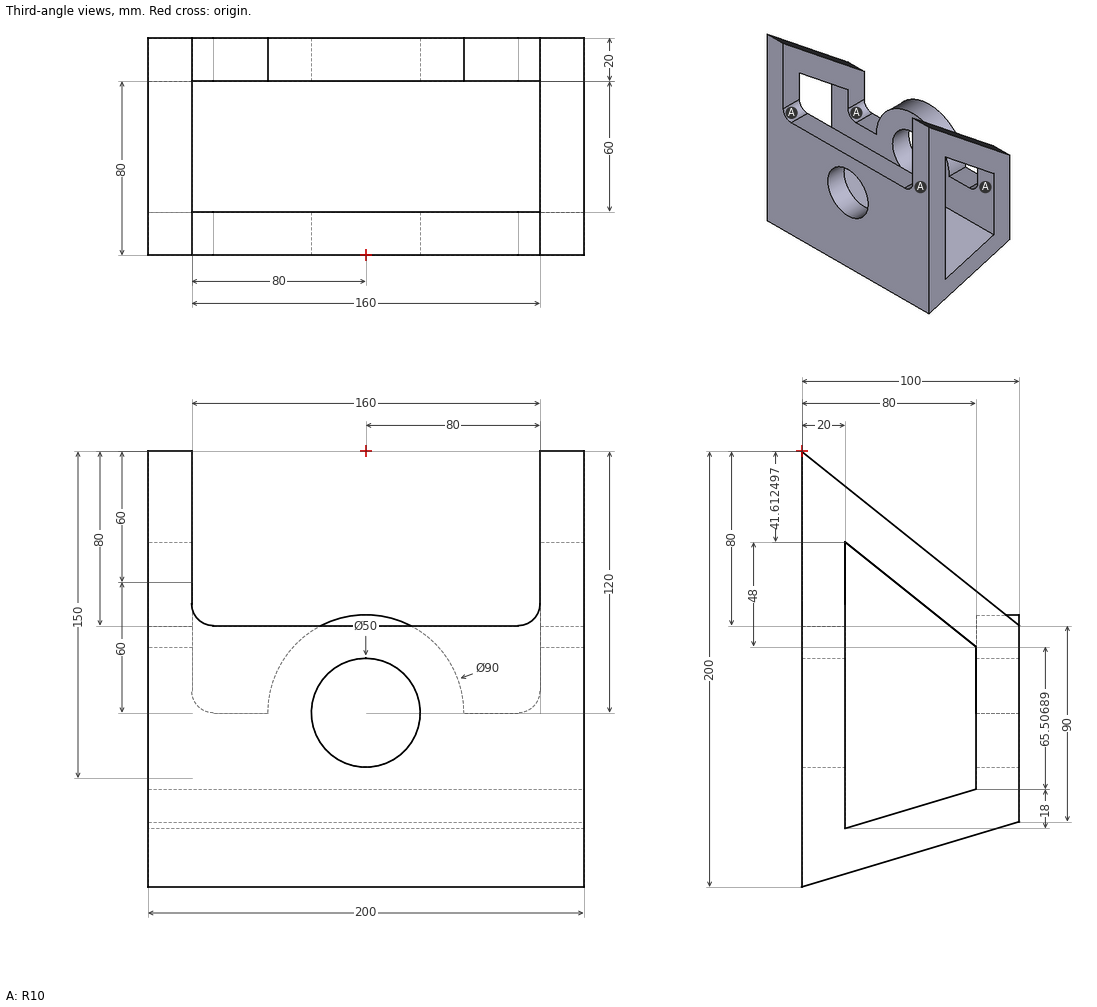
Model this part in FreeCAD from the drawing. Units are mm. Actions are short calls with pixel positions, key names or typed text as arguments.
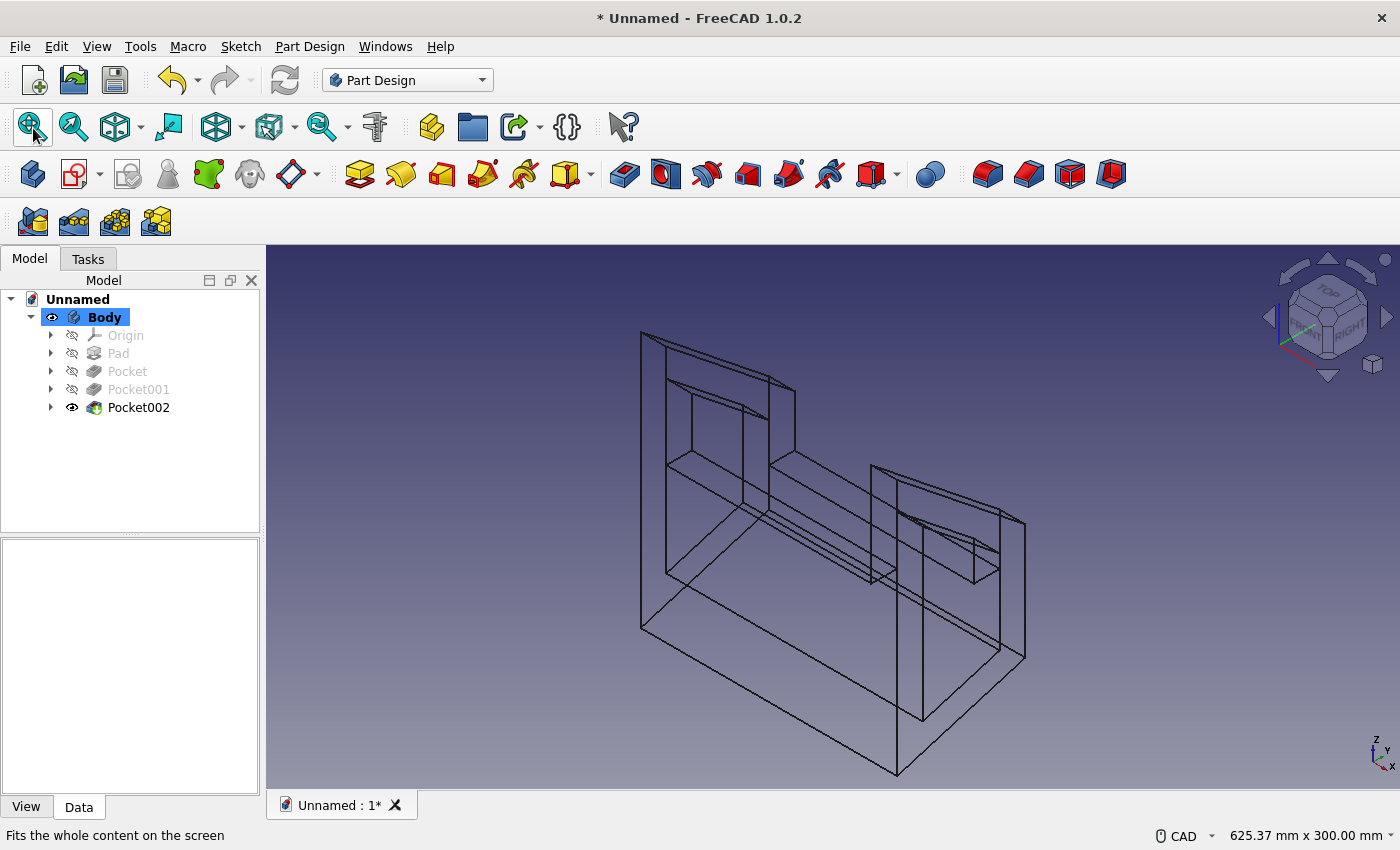
click(987, 575)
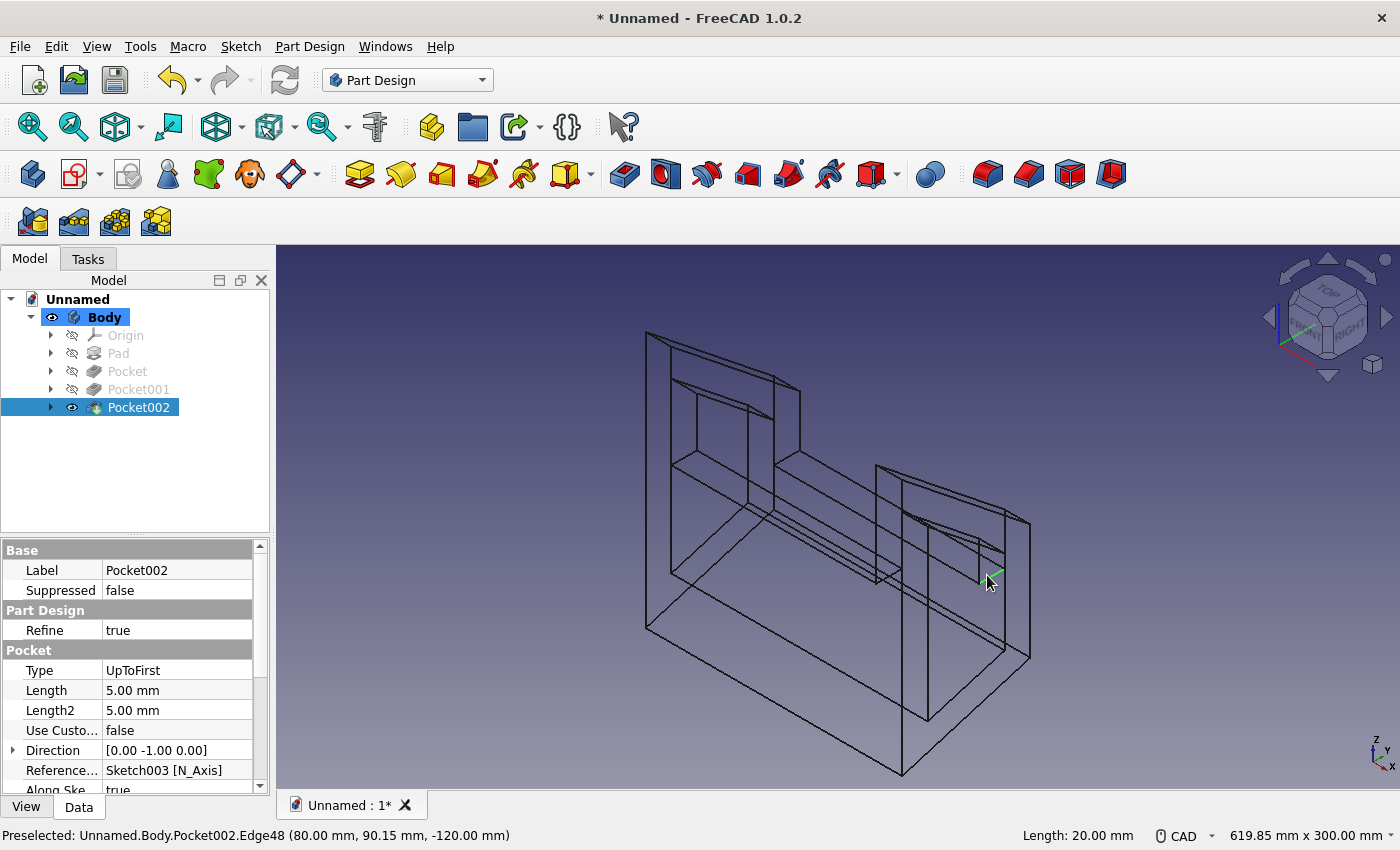
click(787, 457, ctrl)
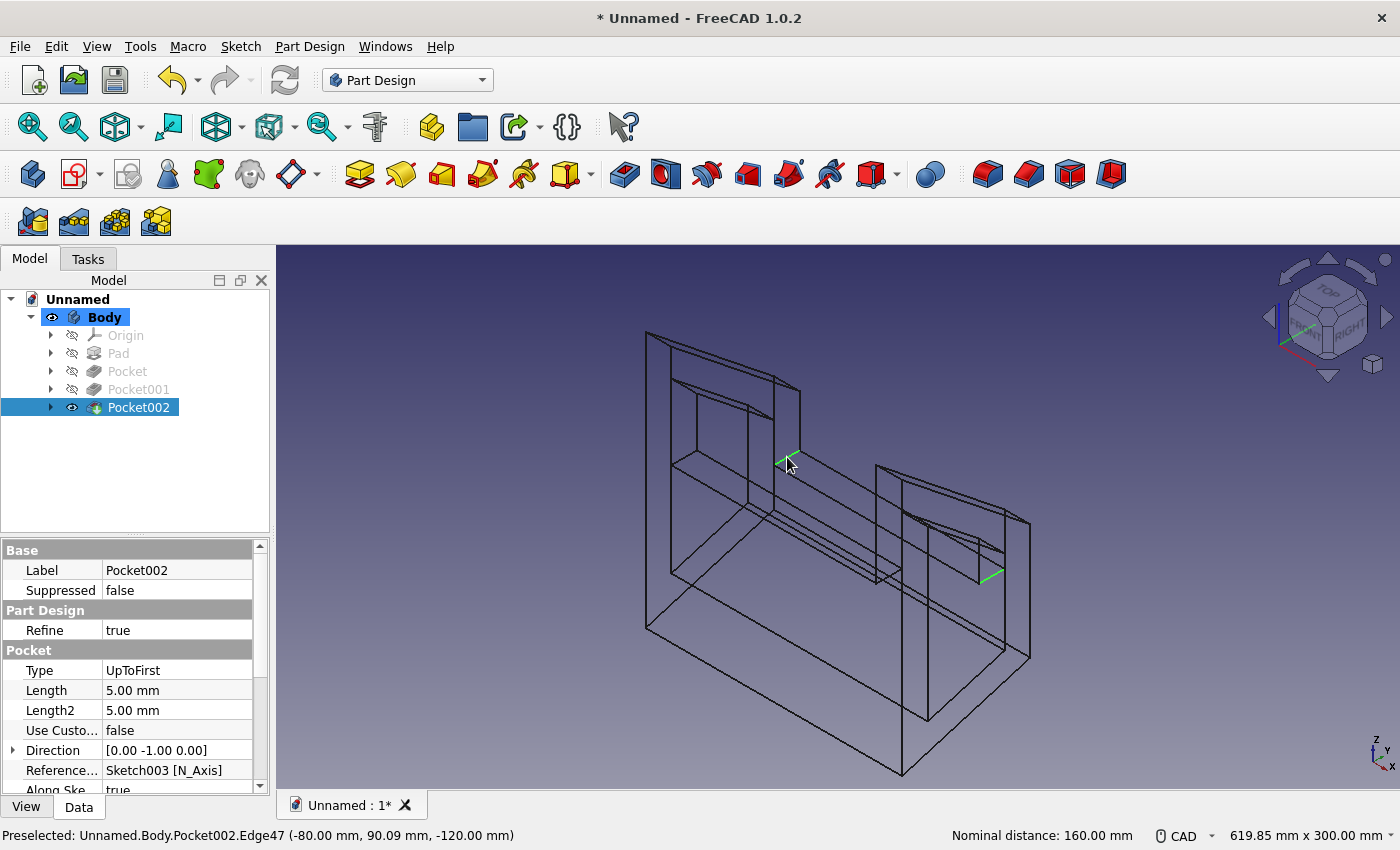
click(684, 457, ctrl)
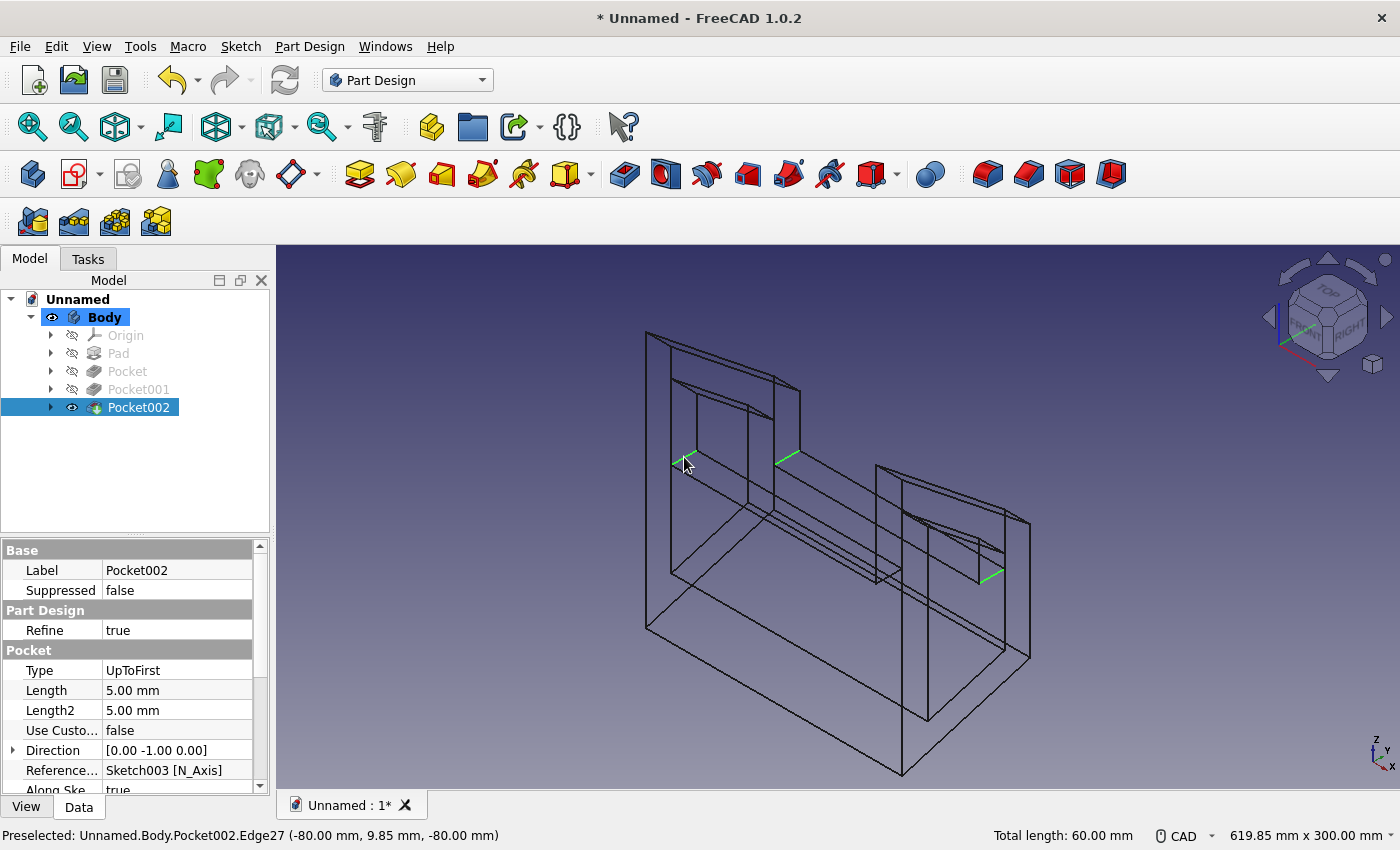
click(889, 575, ctrl)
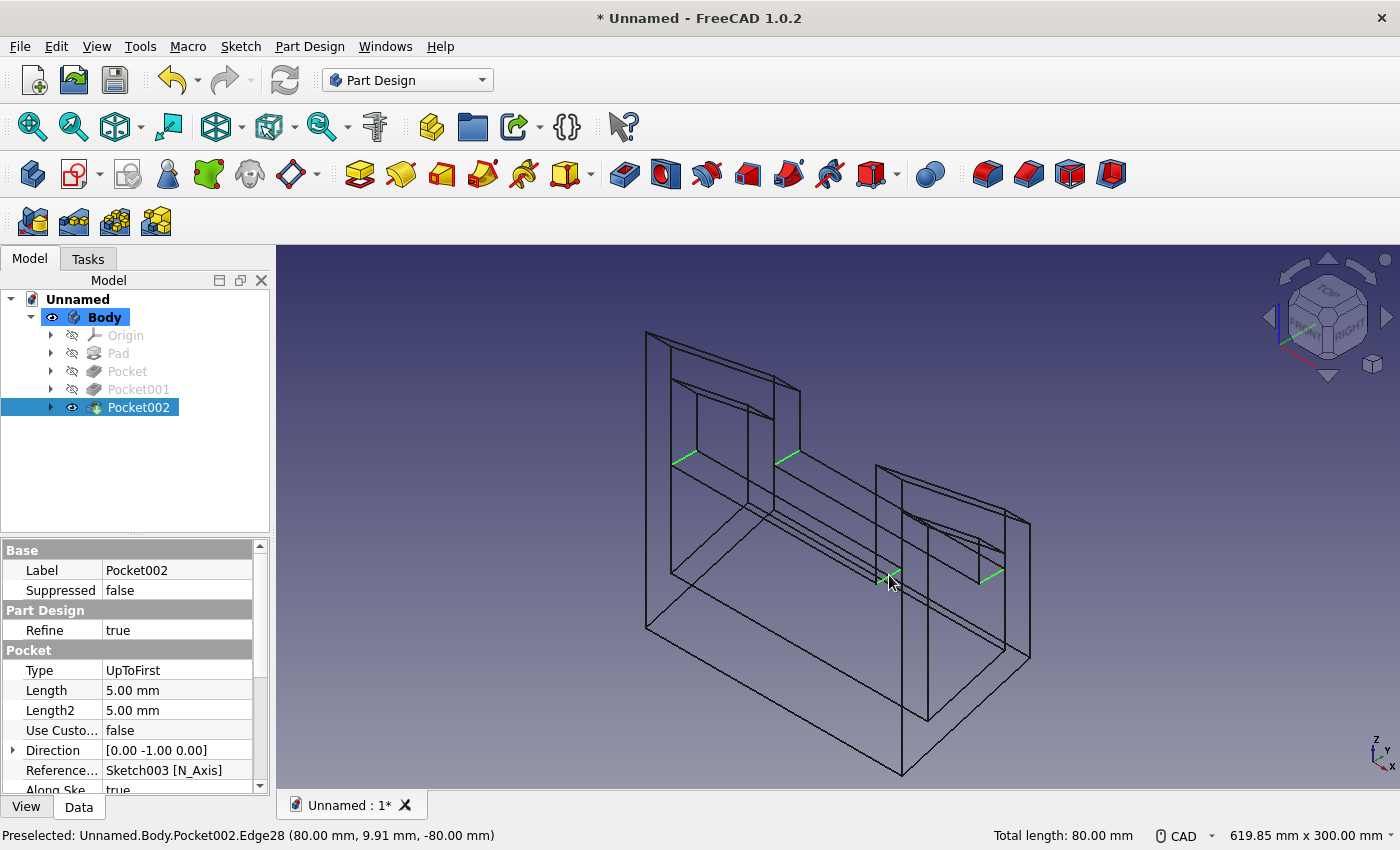
key(v)
key(1)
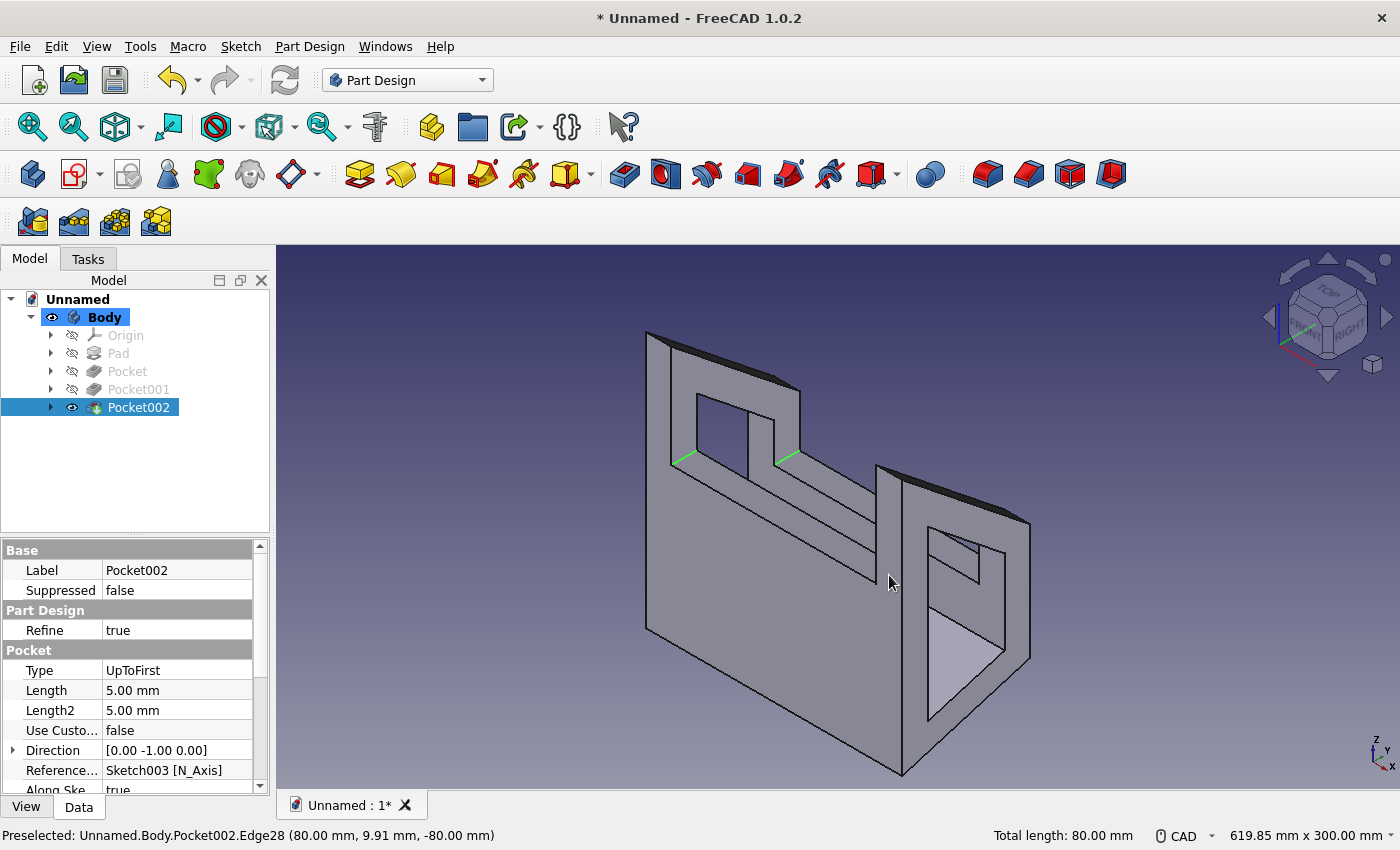
click(988, 174)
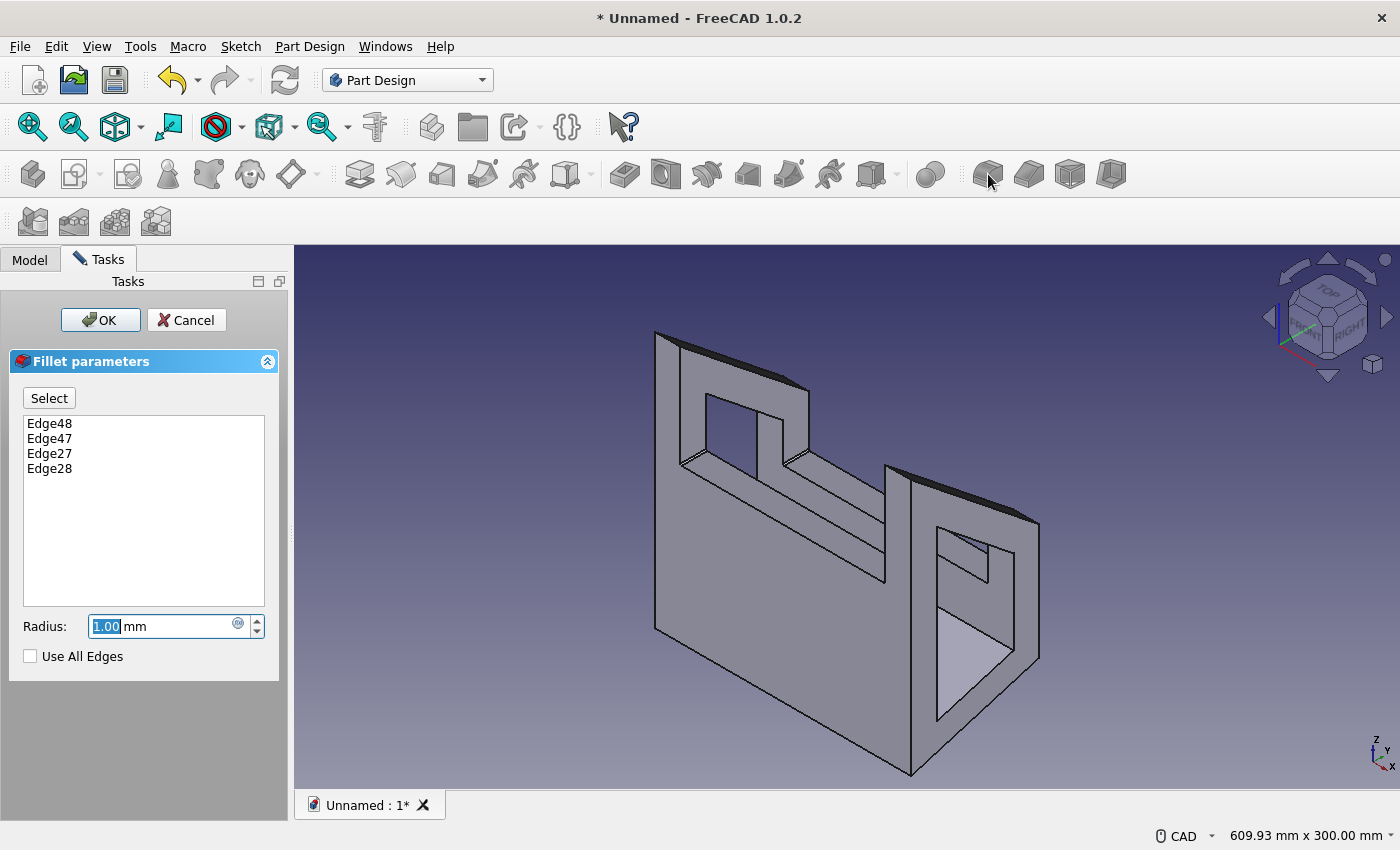
text(10)
key(Tab)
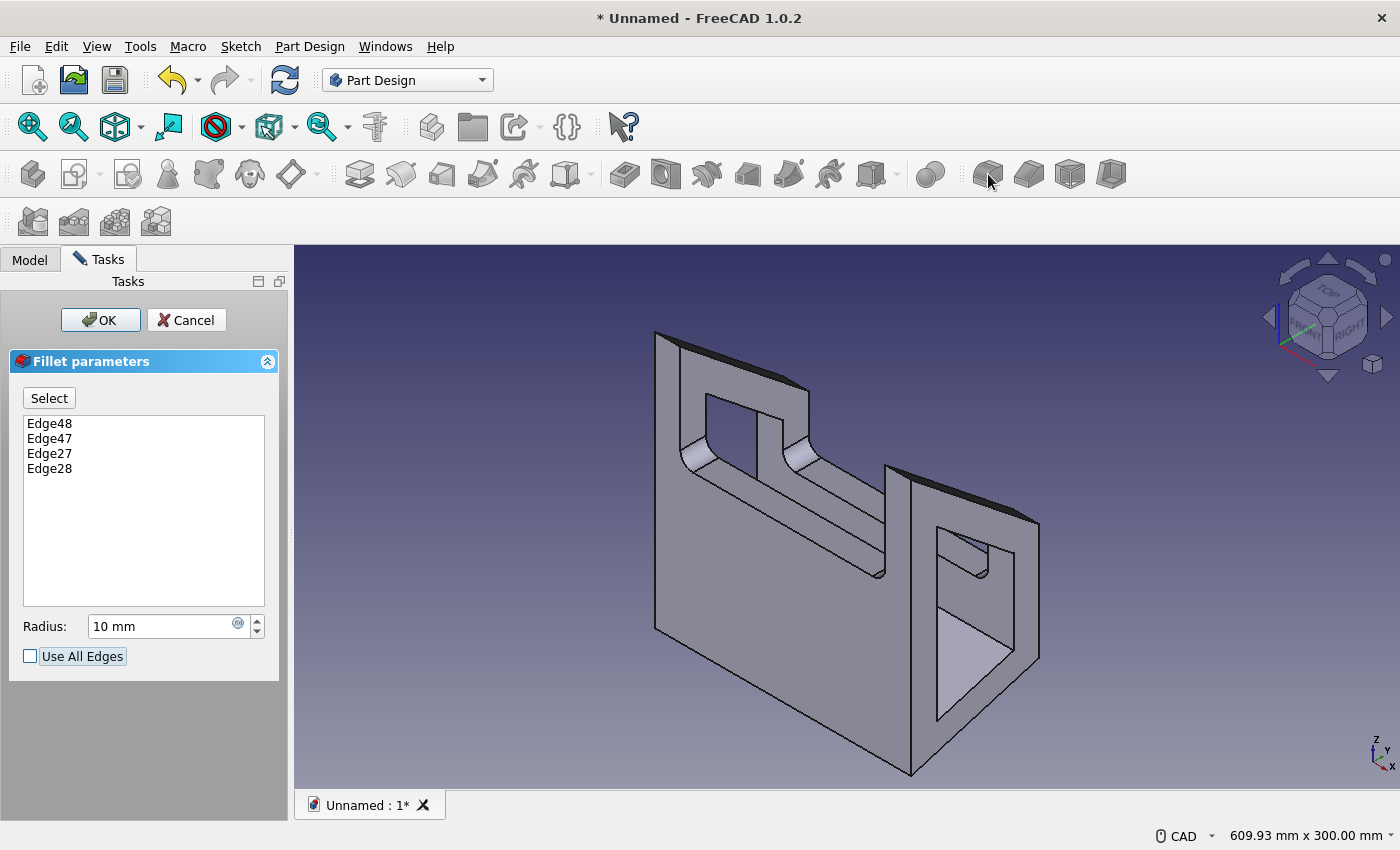
click(101, 320)